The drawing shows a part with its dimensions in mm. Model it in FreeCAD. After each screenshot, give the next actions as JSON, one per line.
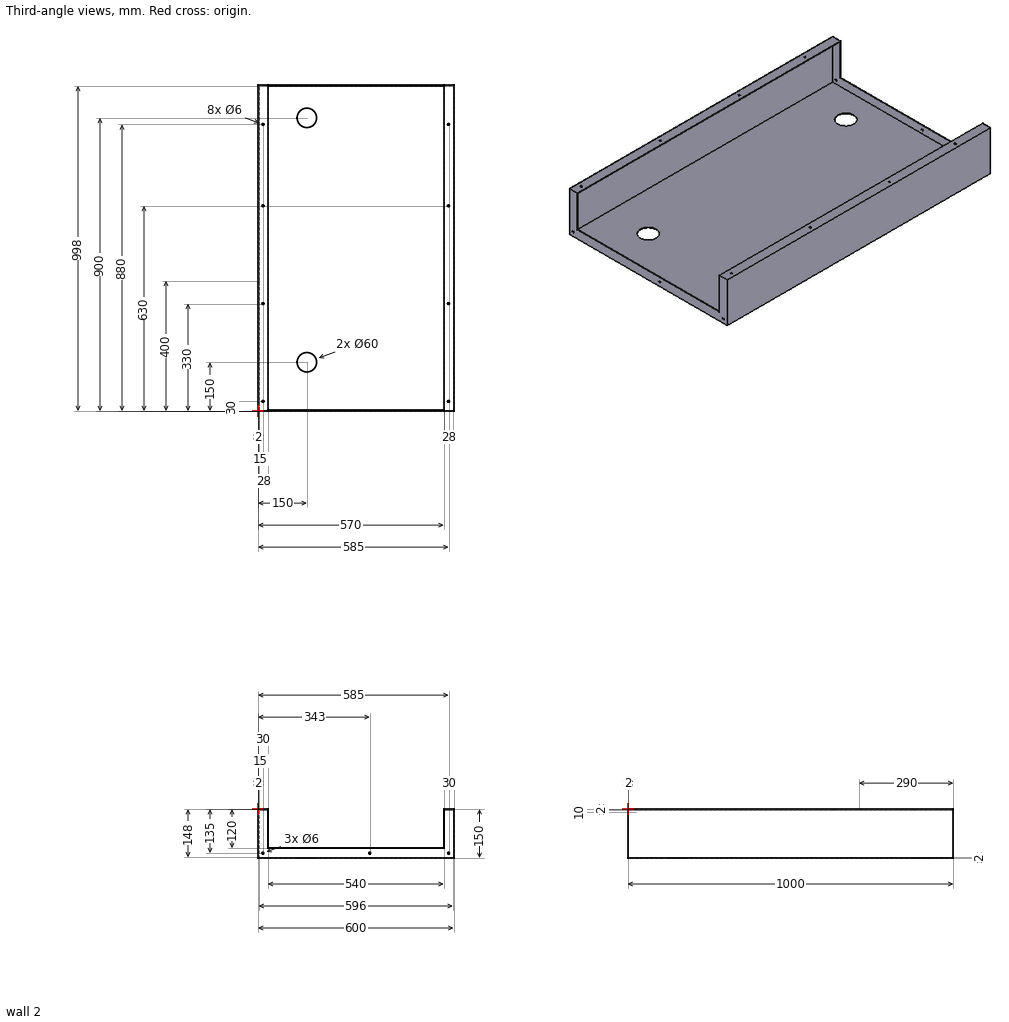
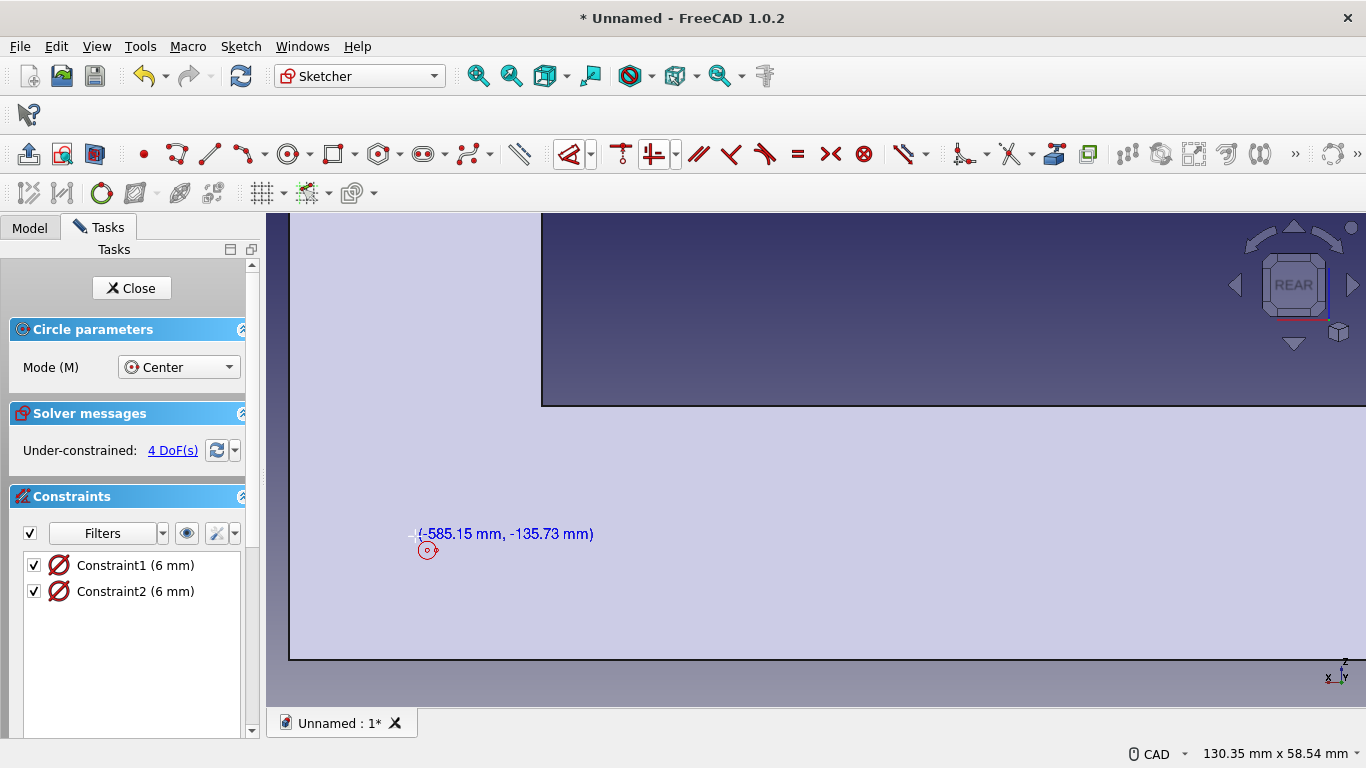
{"action": "scroll", "coordinate": [415, 536], "scroll_direction": "down", "scroll_amount": 10}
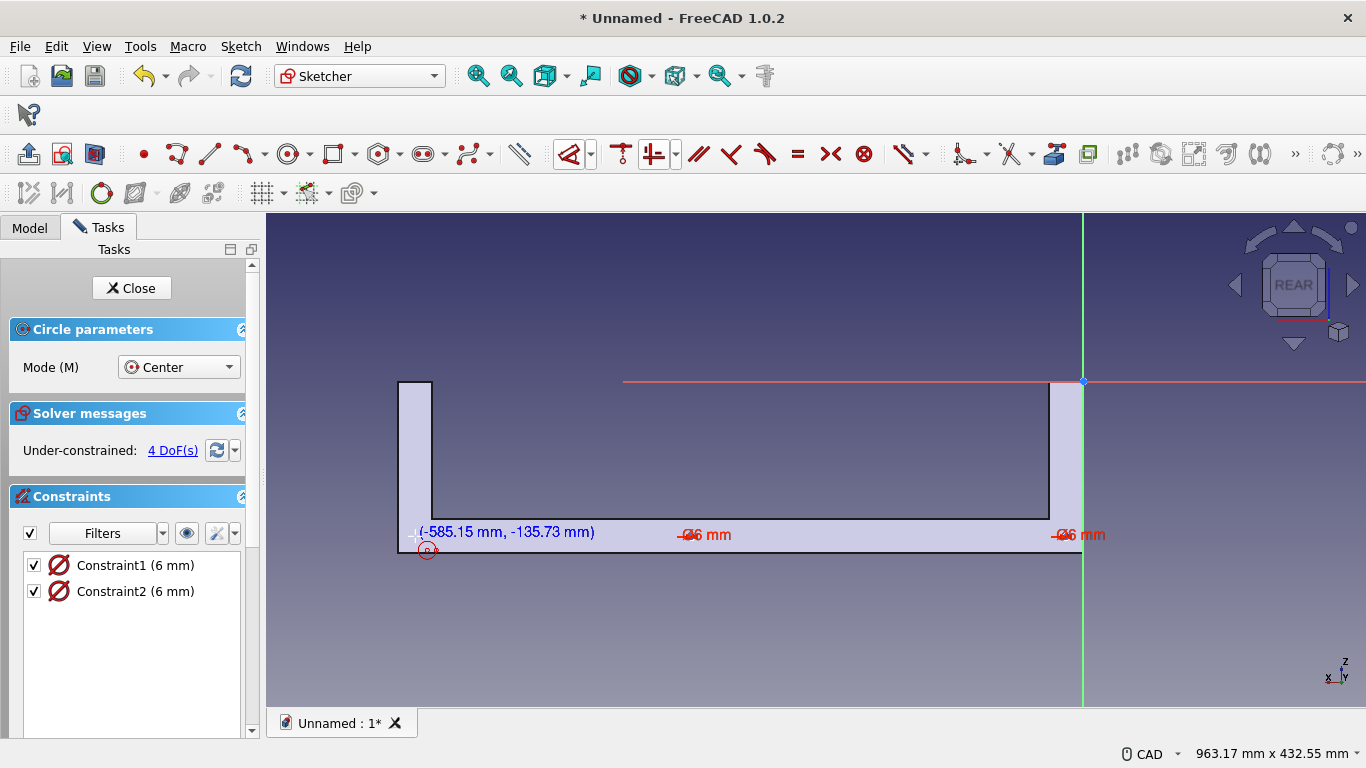
{"action": "left_click", "coordinate": [415, 536]}
{"action": "mouse_move", "coordinate": [418, 534]}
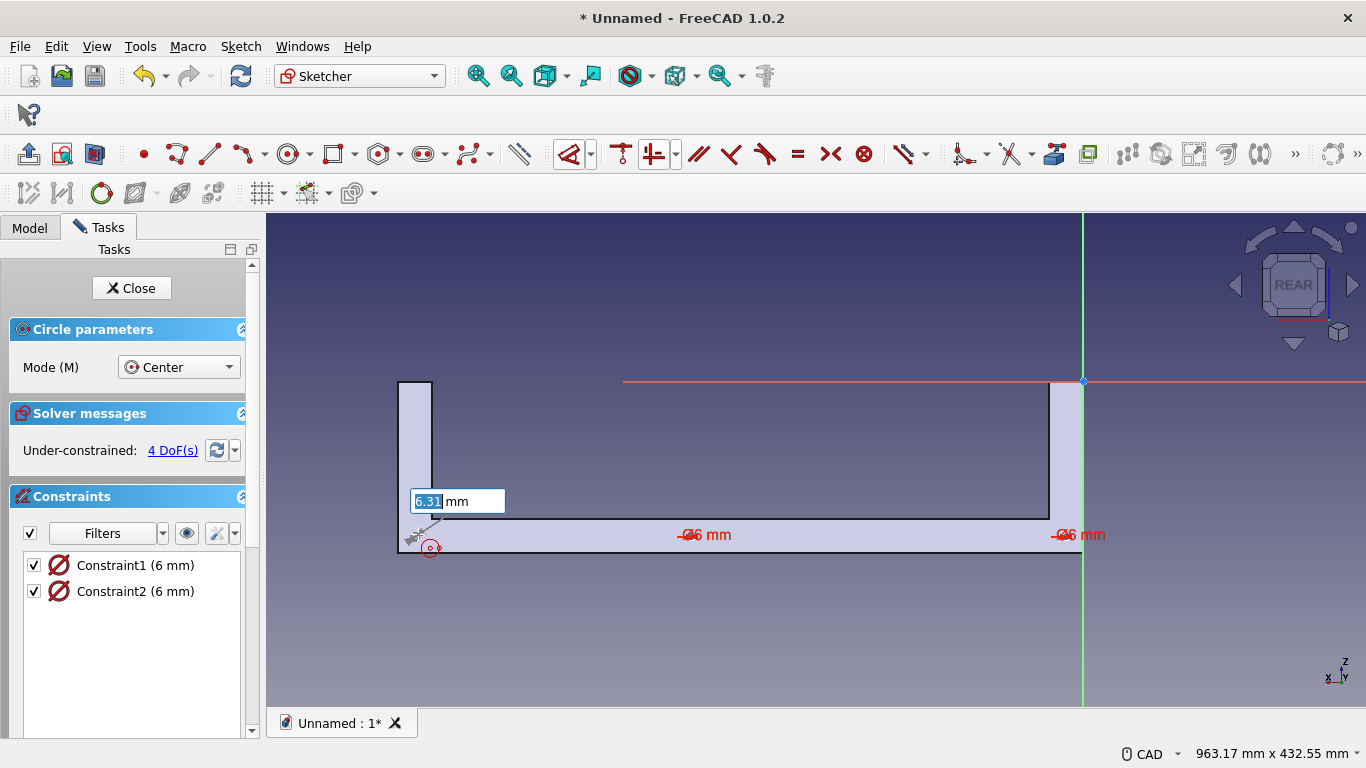
{"action": "type", "text": "6"}
{"action": "key", "text": "Return"}
{"action": "key", "text": "Escape"}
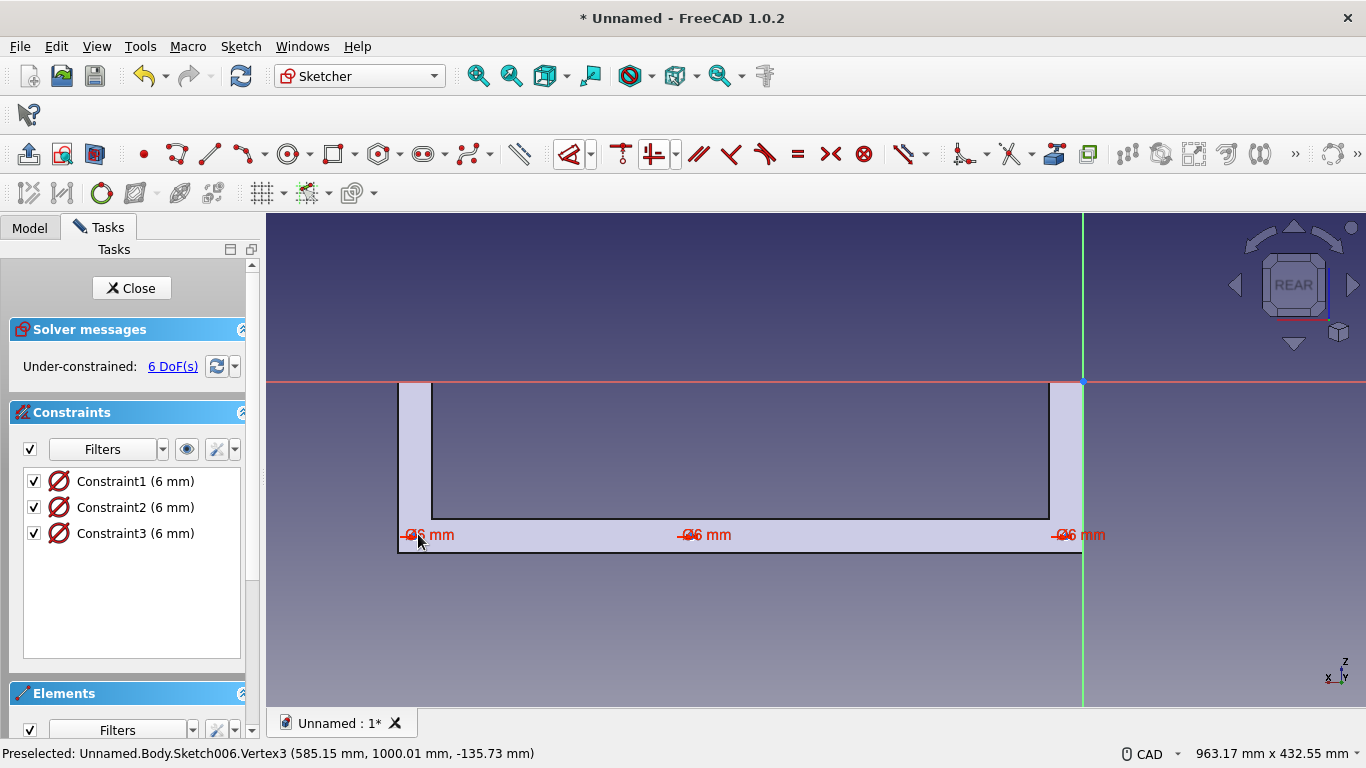
{"action": "scroll", "coordinate": [1066, 537], "scroll_direction": "up", "scroll_amount": 5}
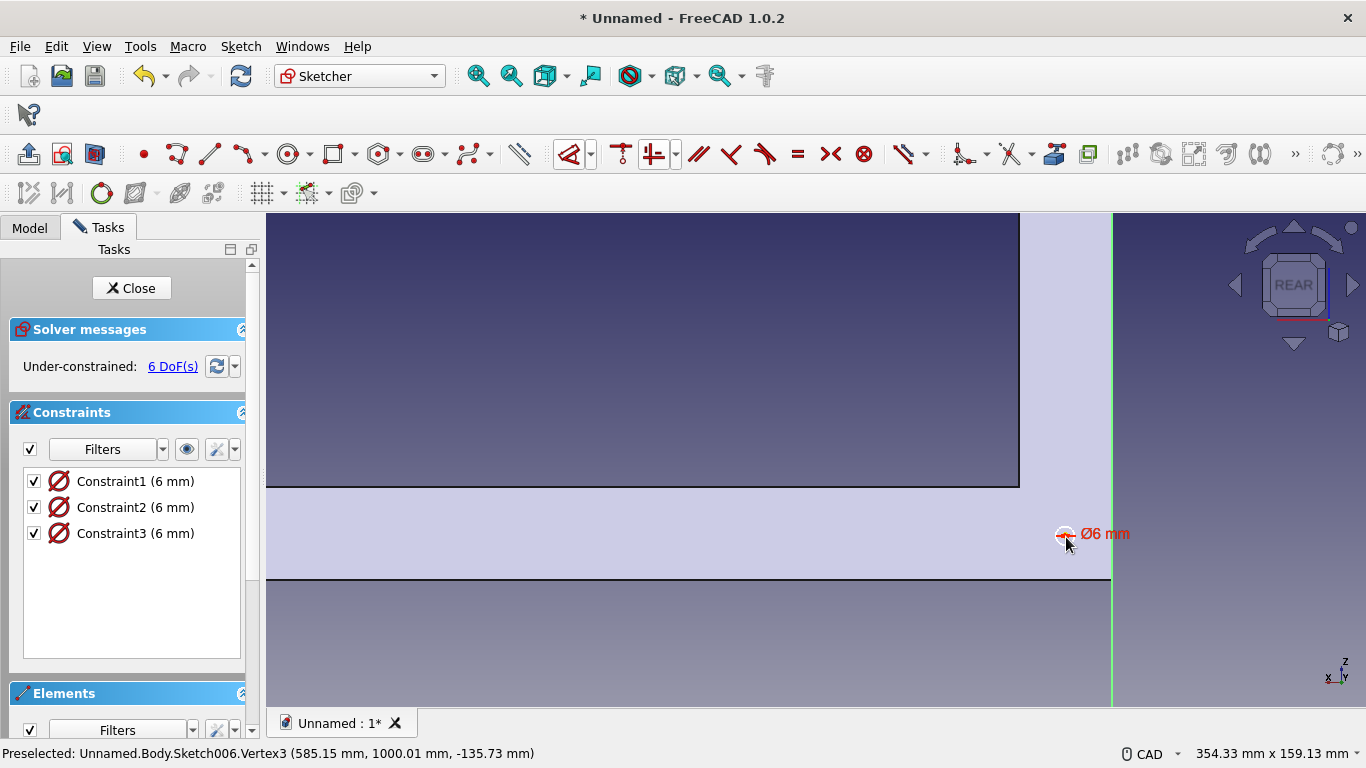
{"action": "left_click", "coordinate": [1065, 536]}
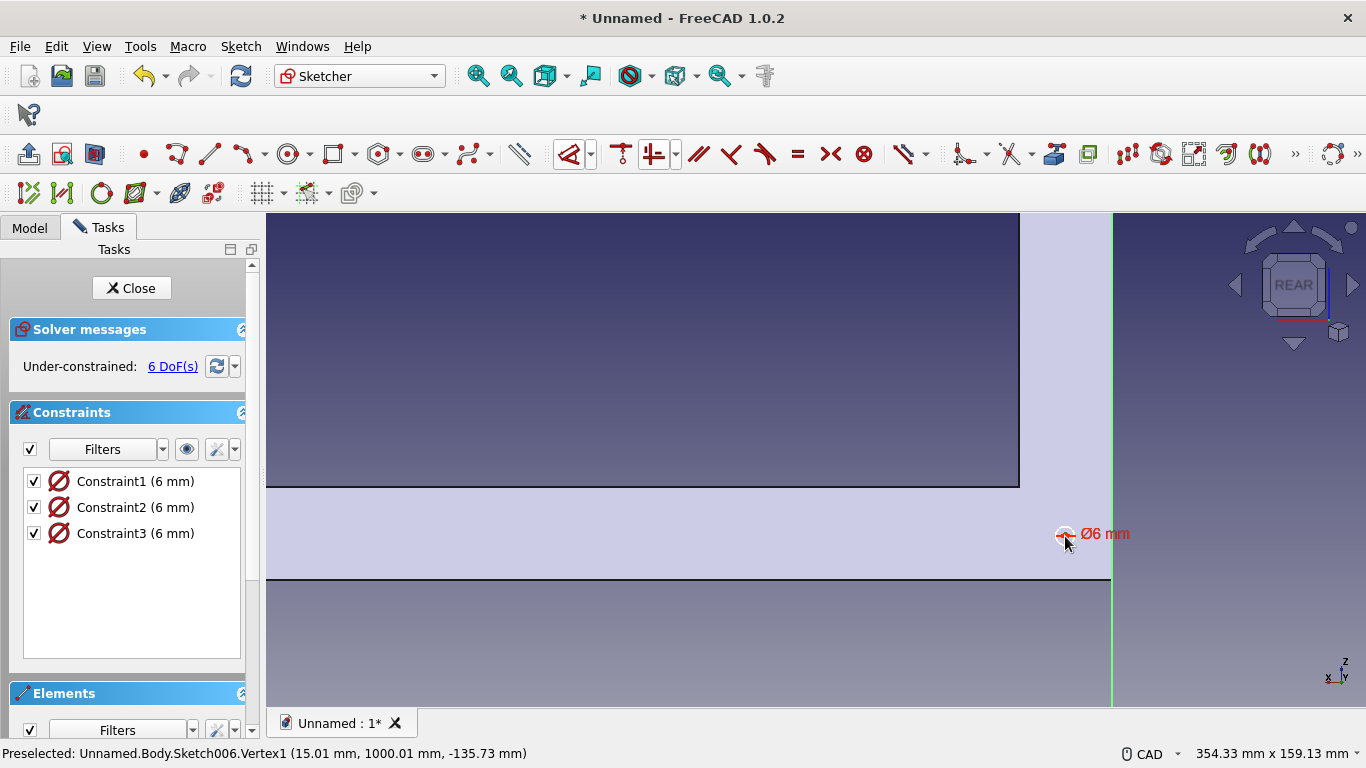
{"action": "left_click", "coordinate": [590, 154]}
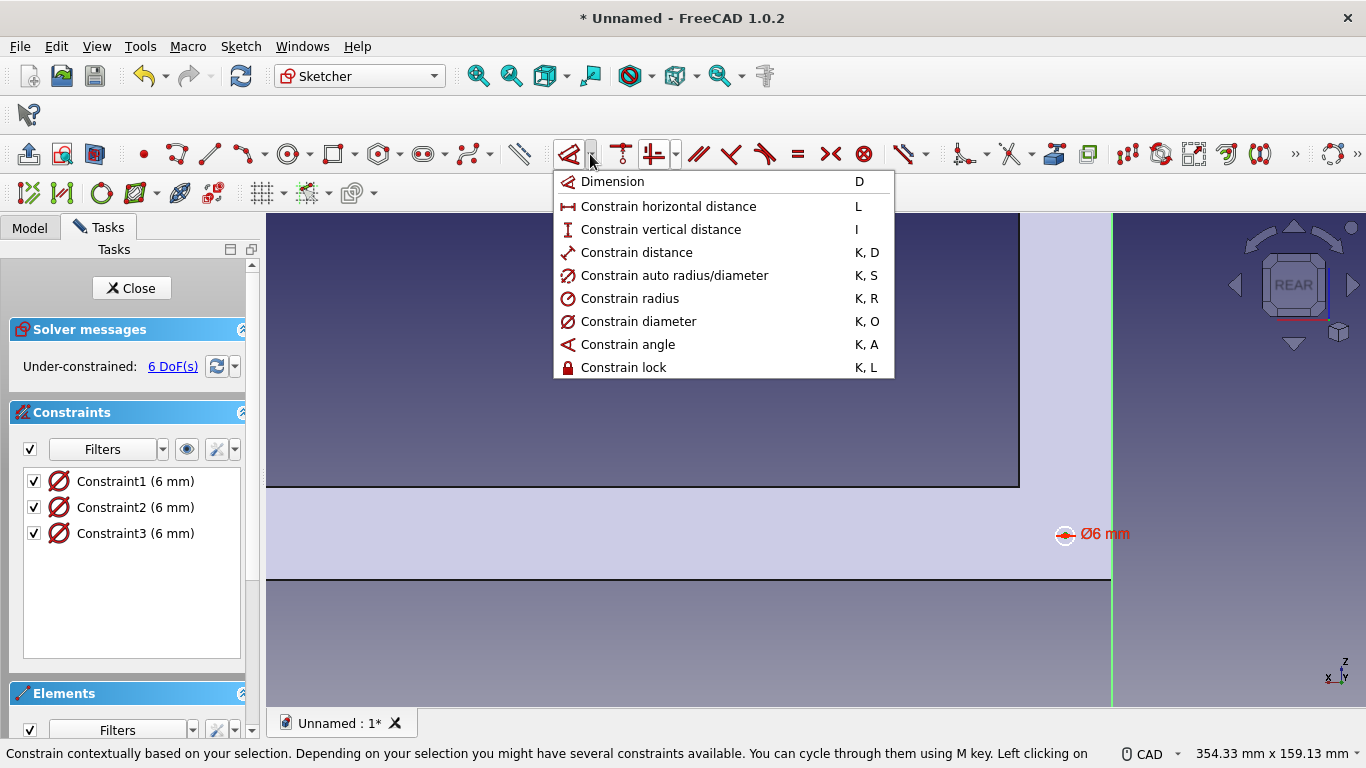
{"action": "left_click", "coordinate": [724, 206]}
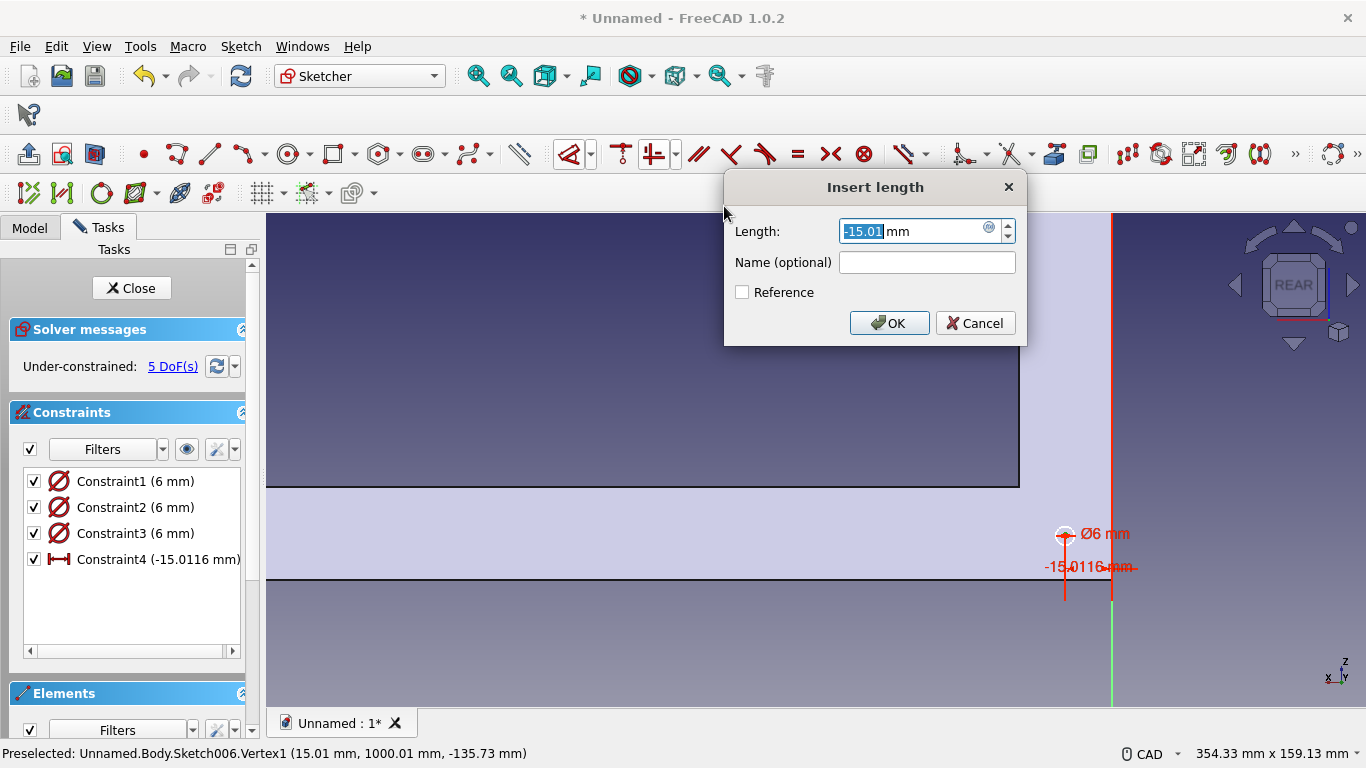
{"action": "type", "text": "-15"}
{"action": "key", "text": "Return"}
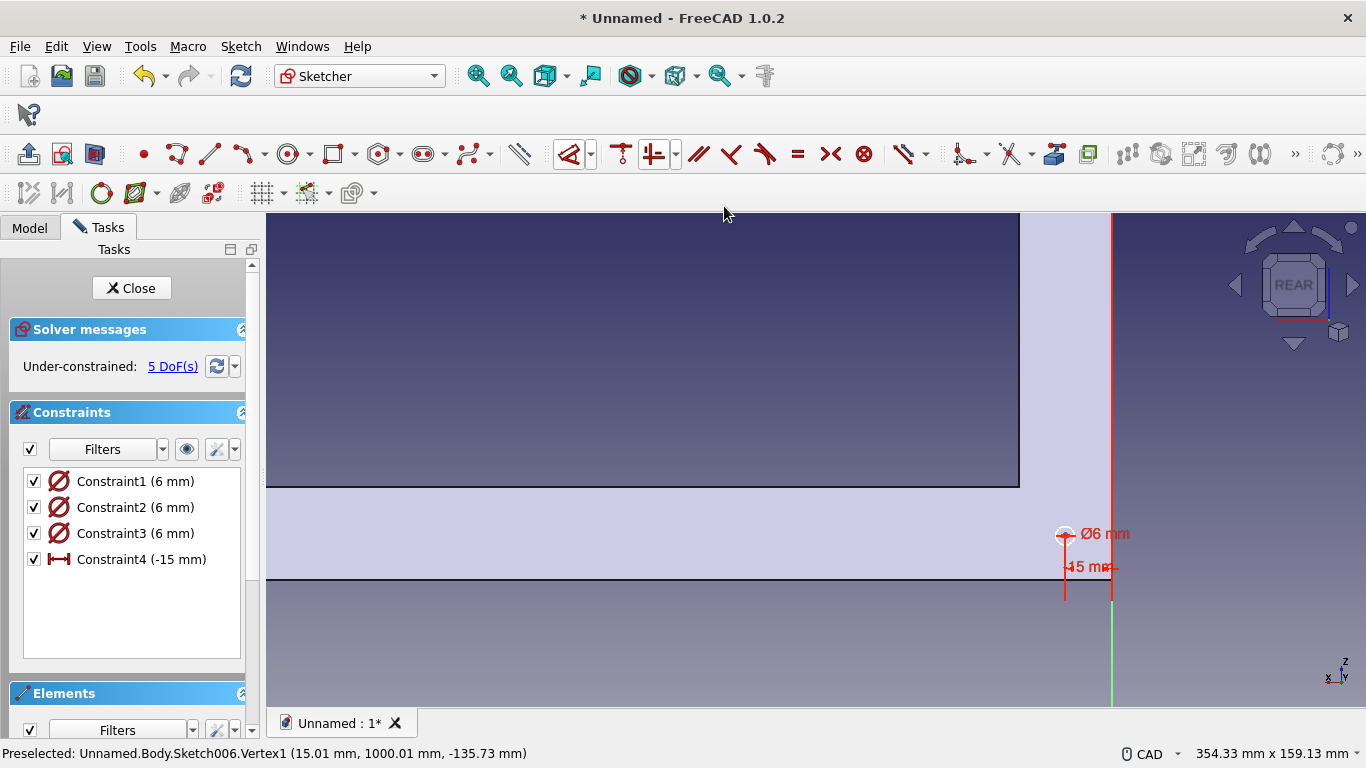
{"action": "left_click", "coordinate": [1065, 536]}